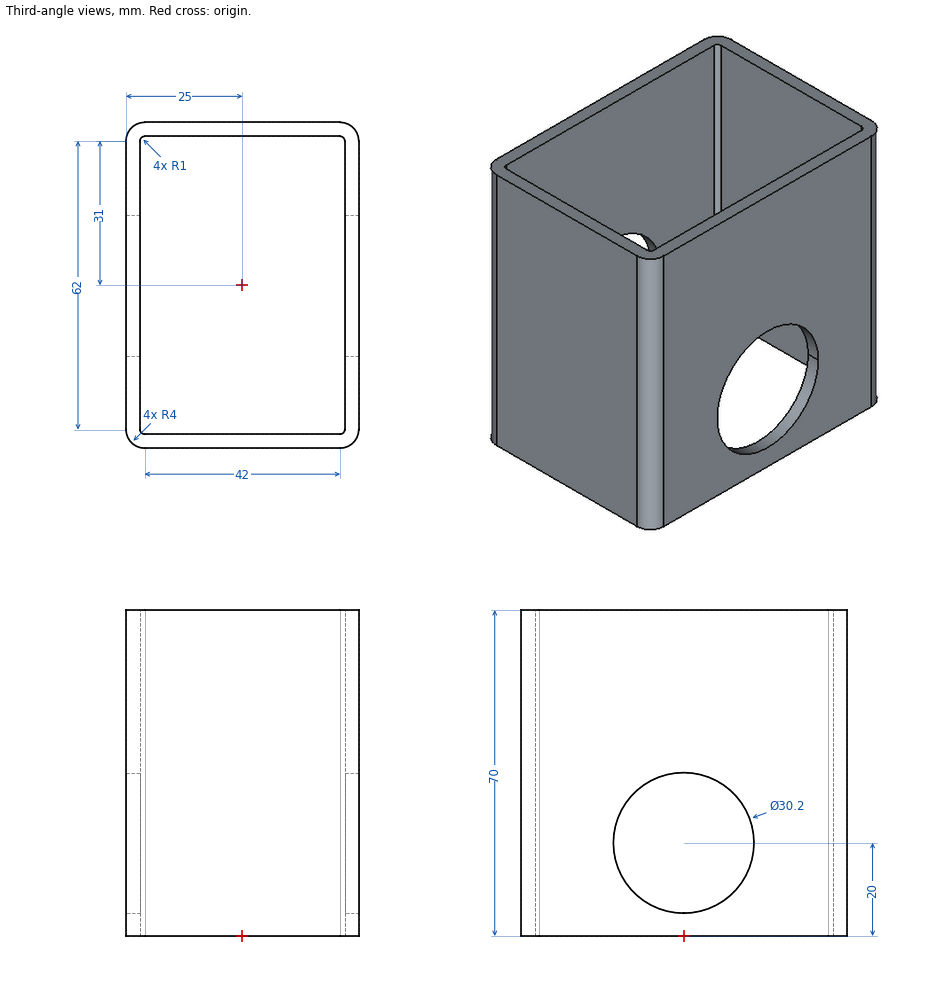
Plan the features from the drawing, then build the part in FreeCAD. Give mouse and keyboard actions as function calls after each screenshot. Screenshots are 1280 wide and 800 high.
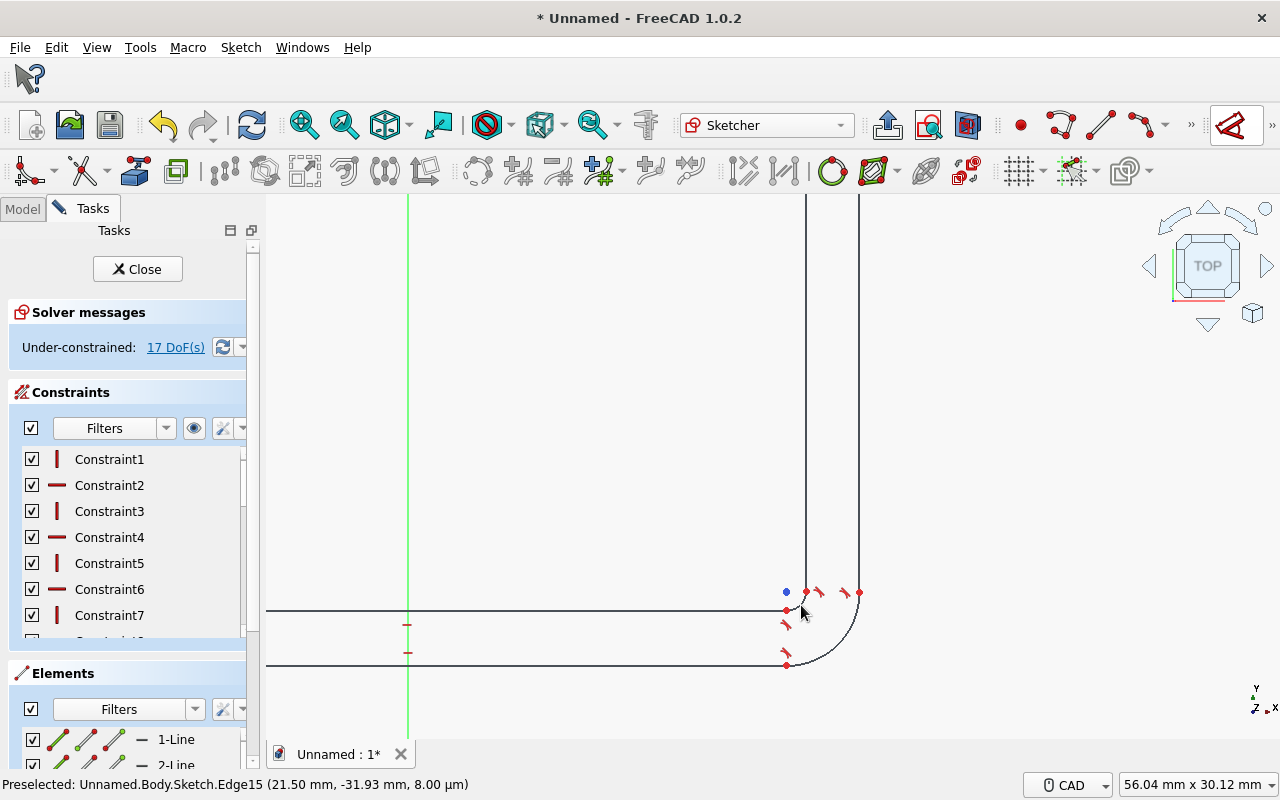
click(559, 611)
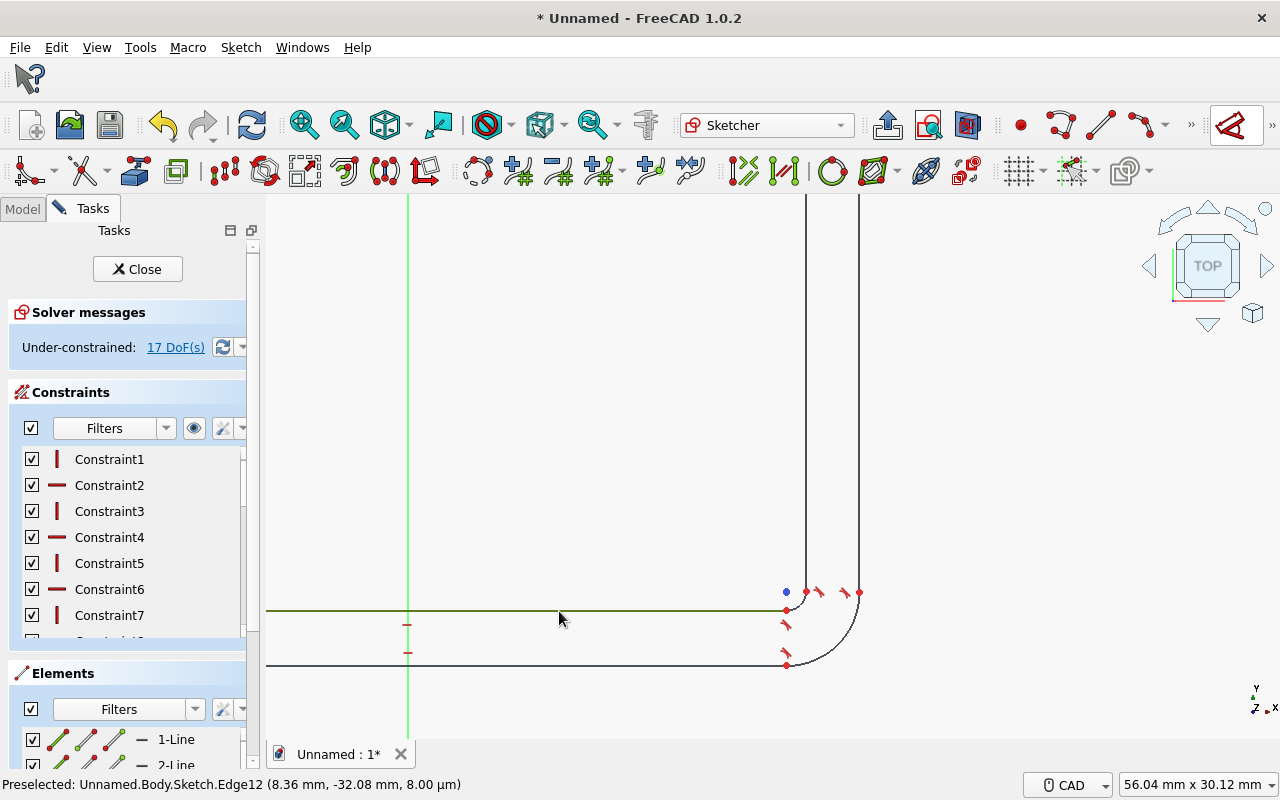
scroll(802, 609, down, 7)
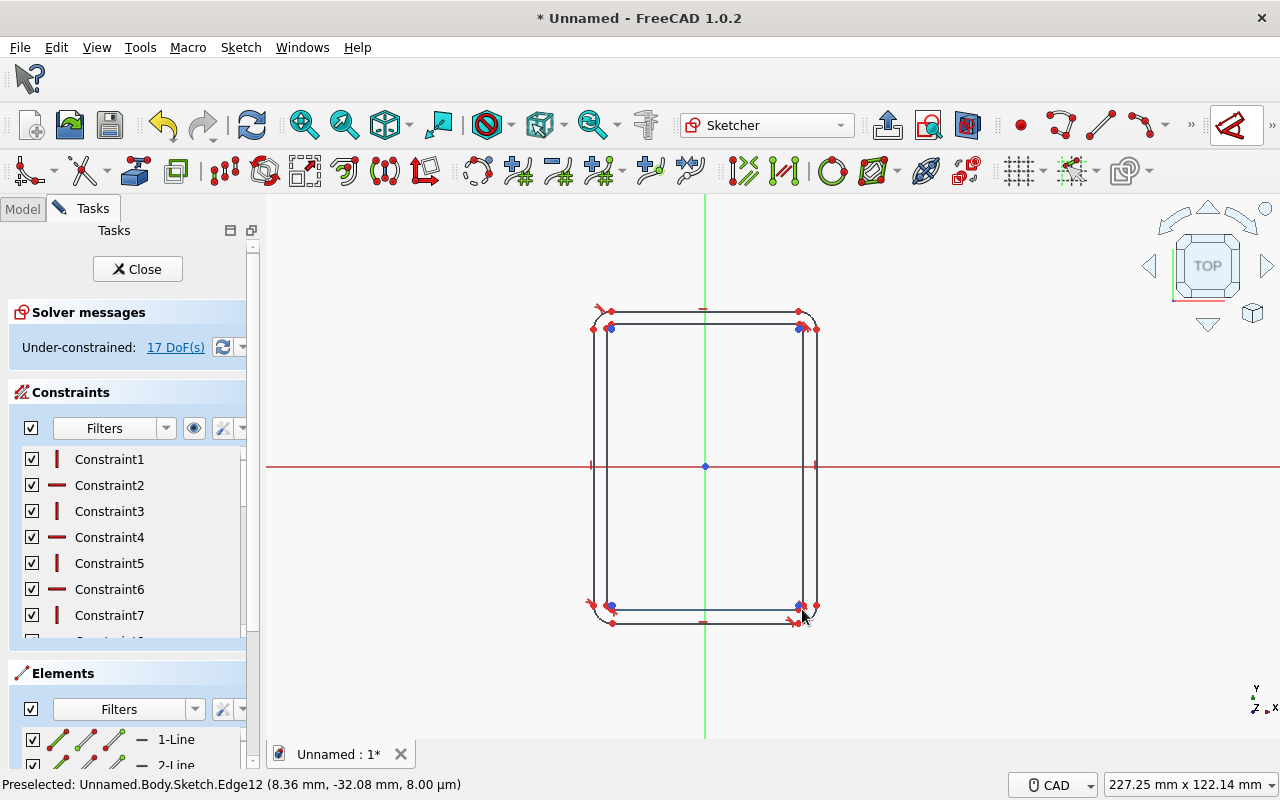
scroll(607, 607, up, 10)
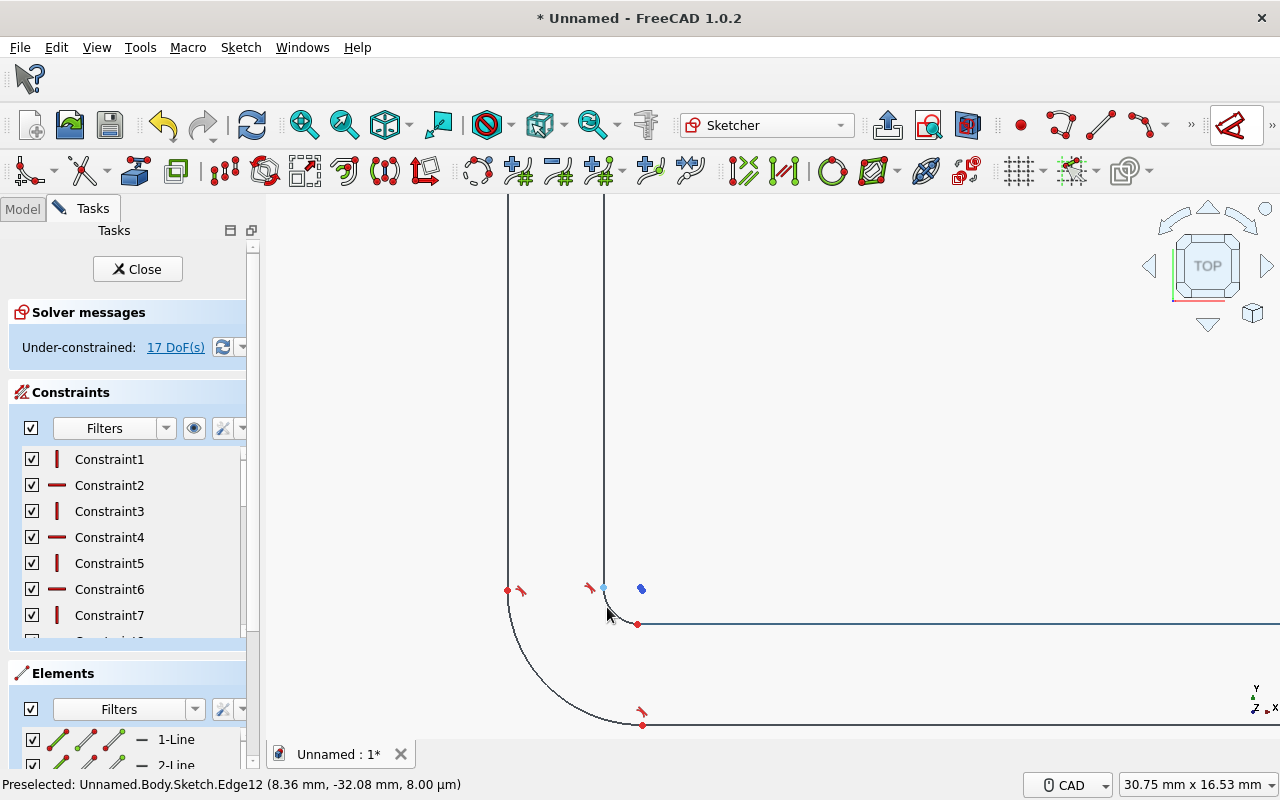
click(607, 603)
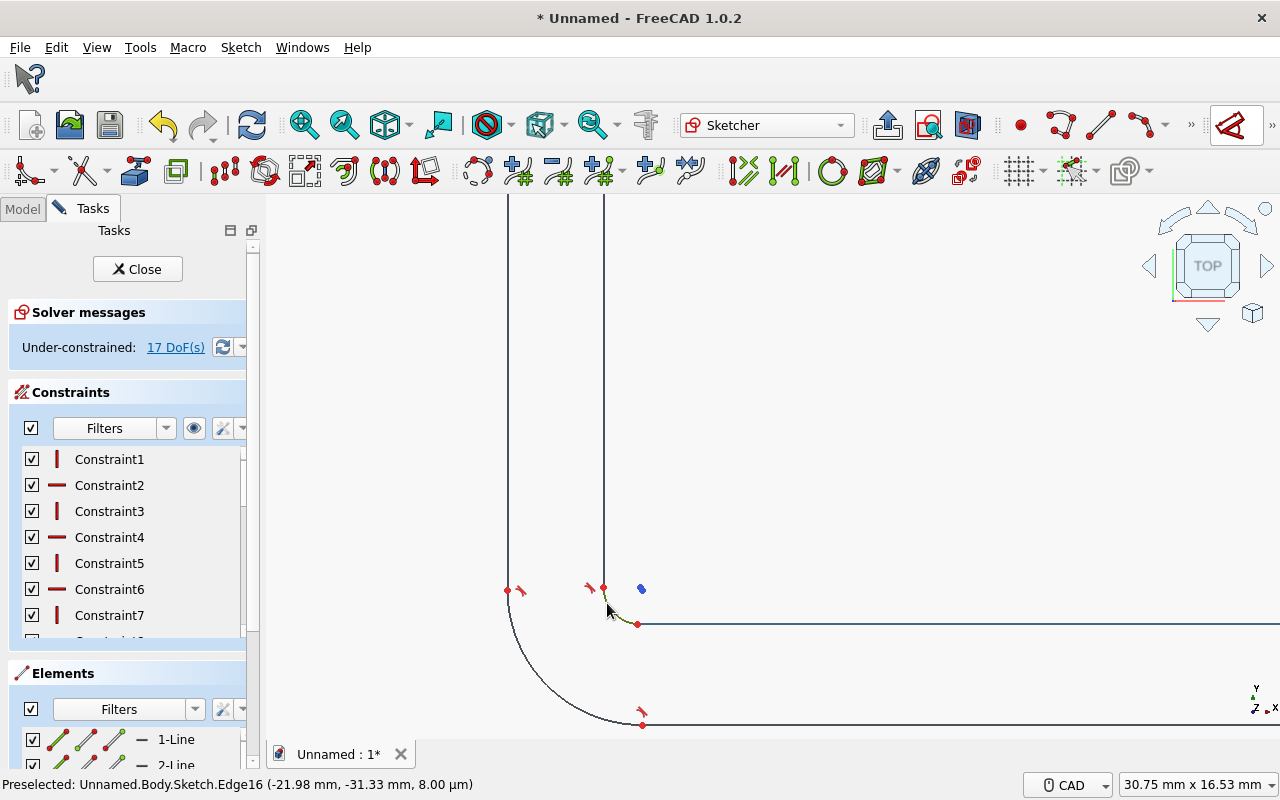
key(t)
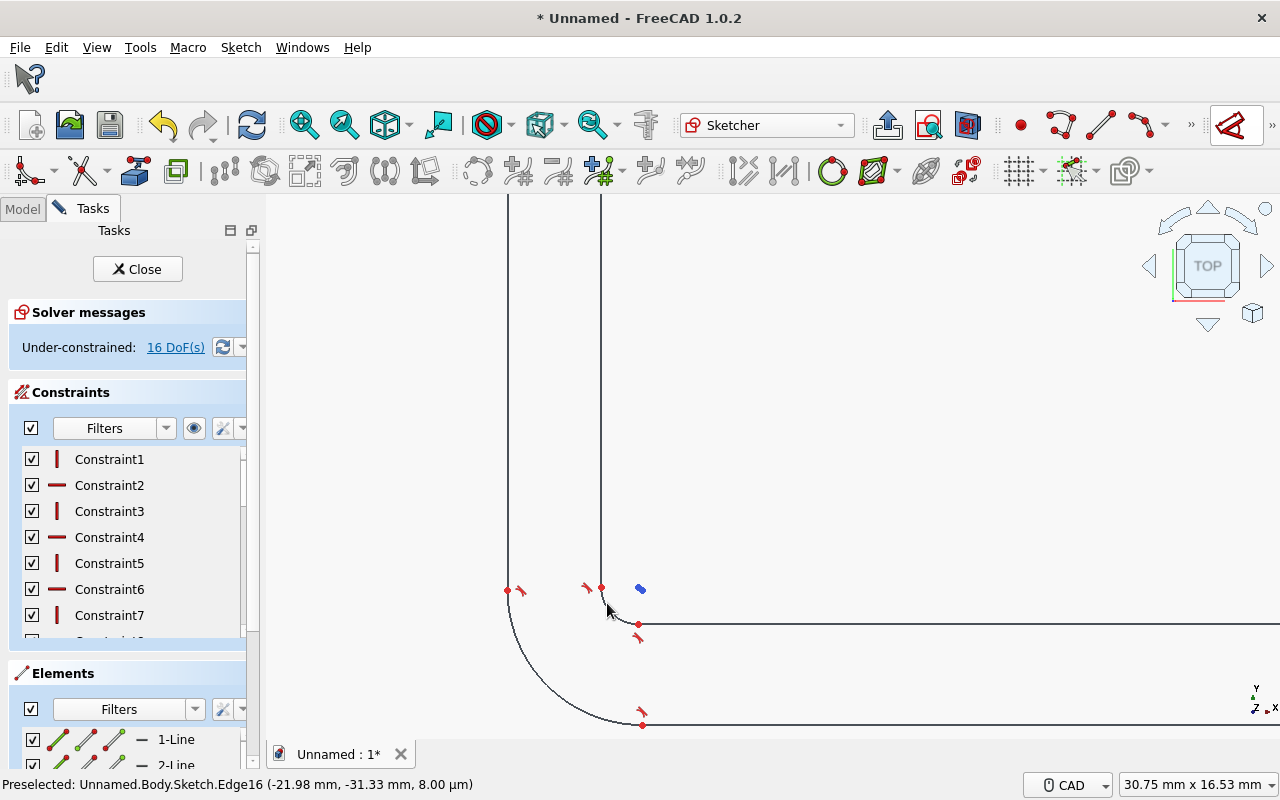
scroll(607, 607, down, 10)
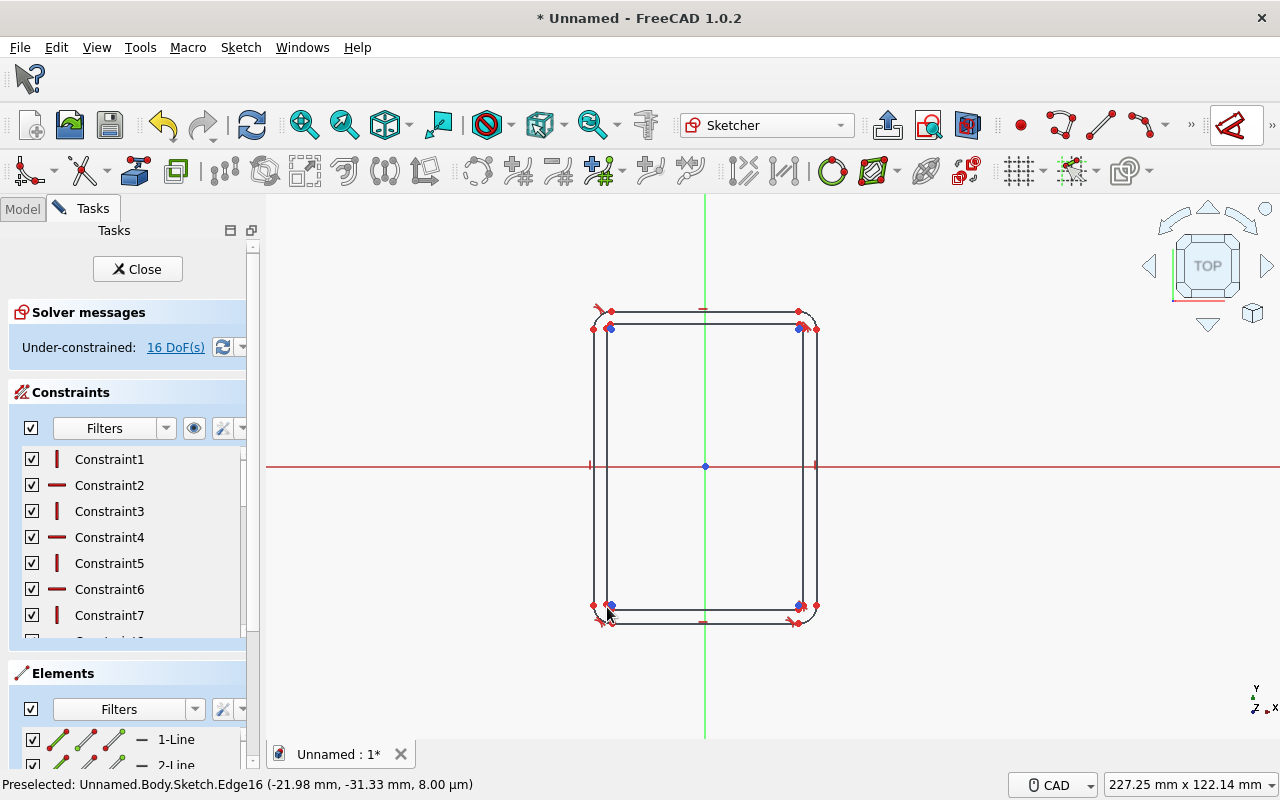
scroll(604, 314, up, 3)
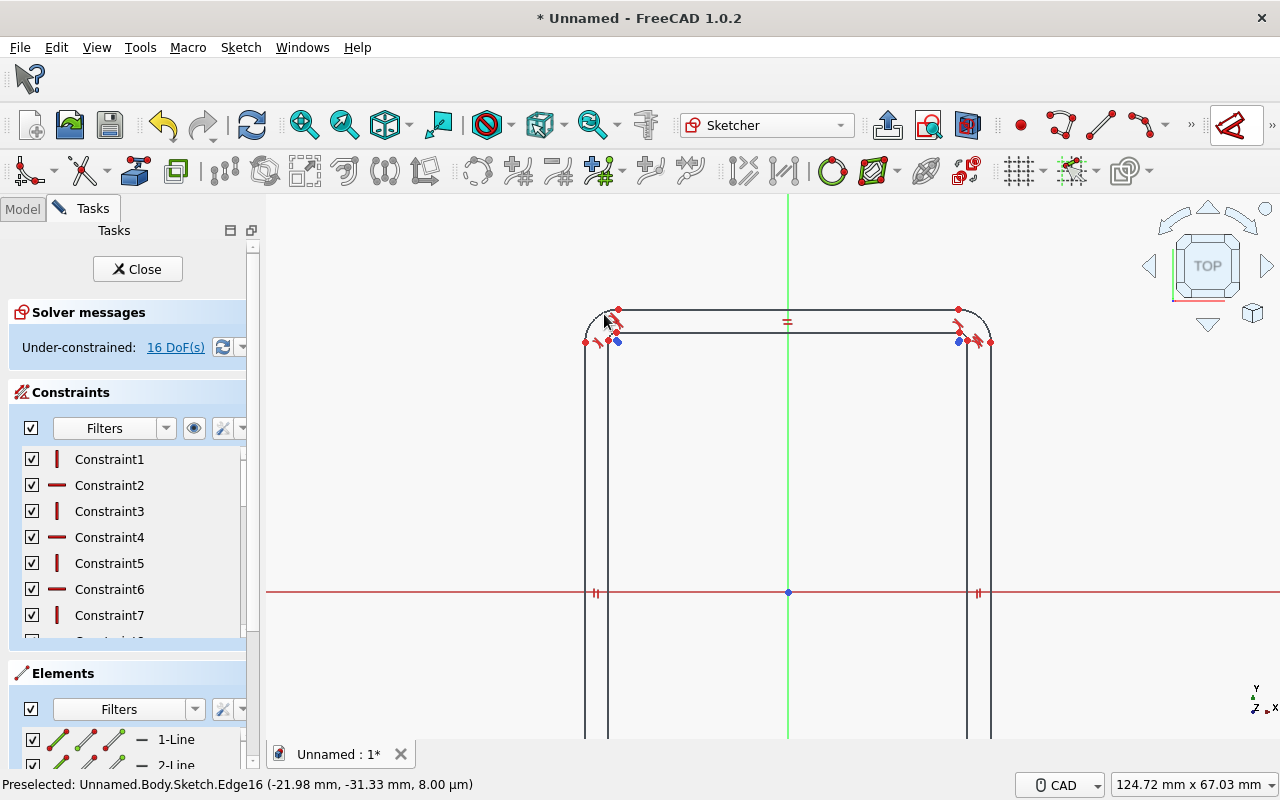
click(603, 313)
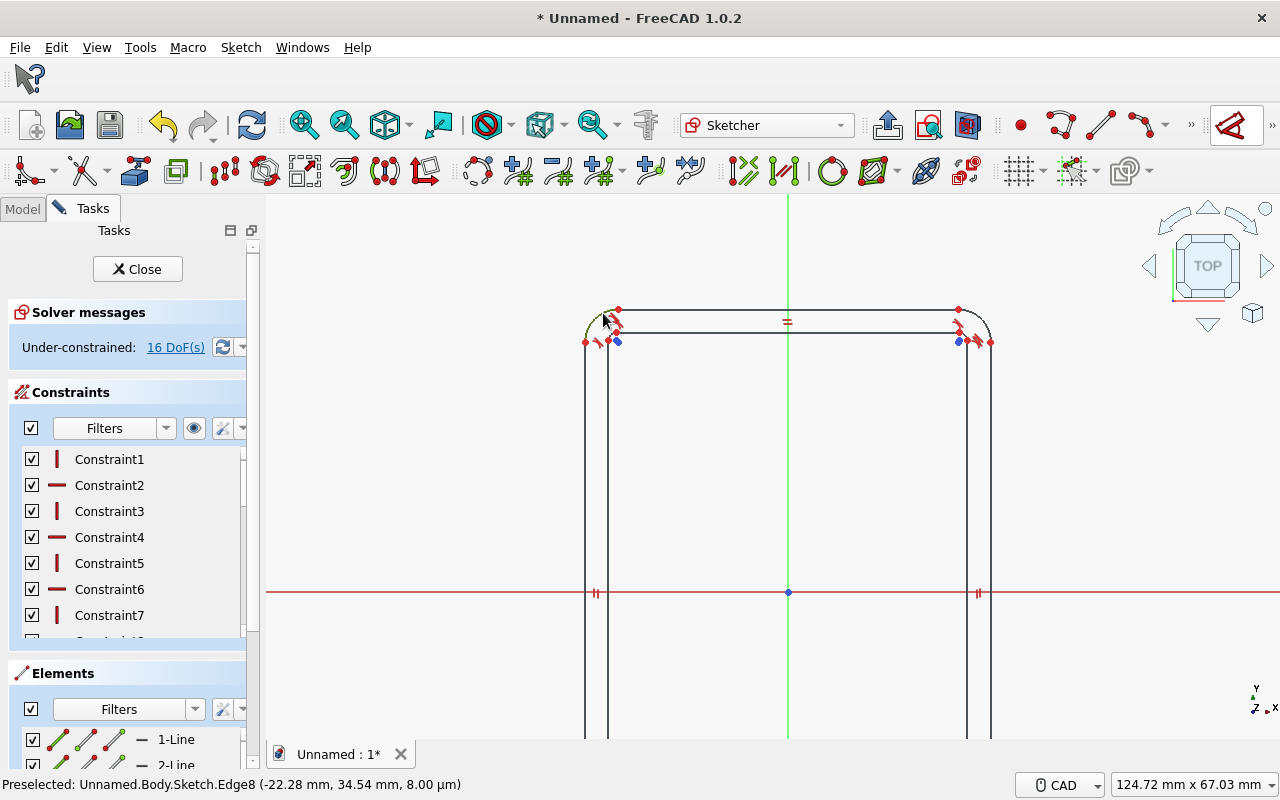
scroll(611, 335, up, 5)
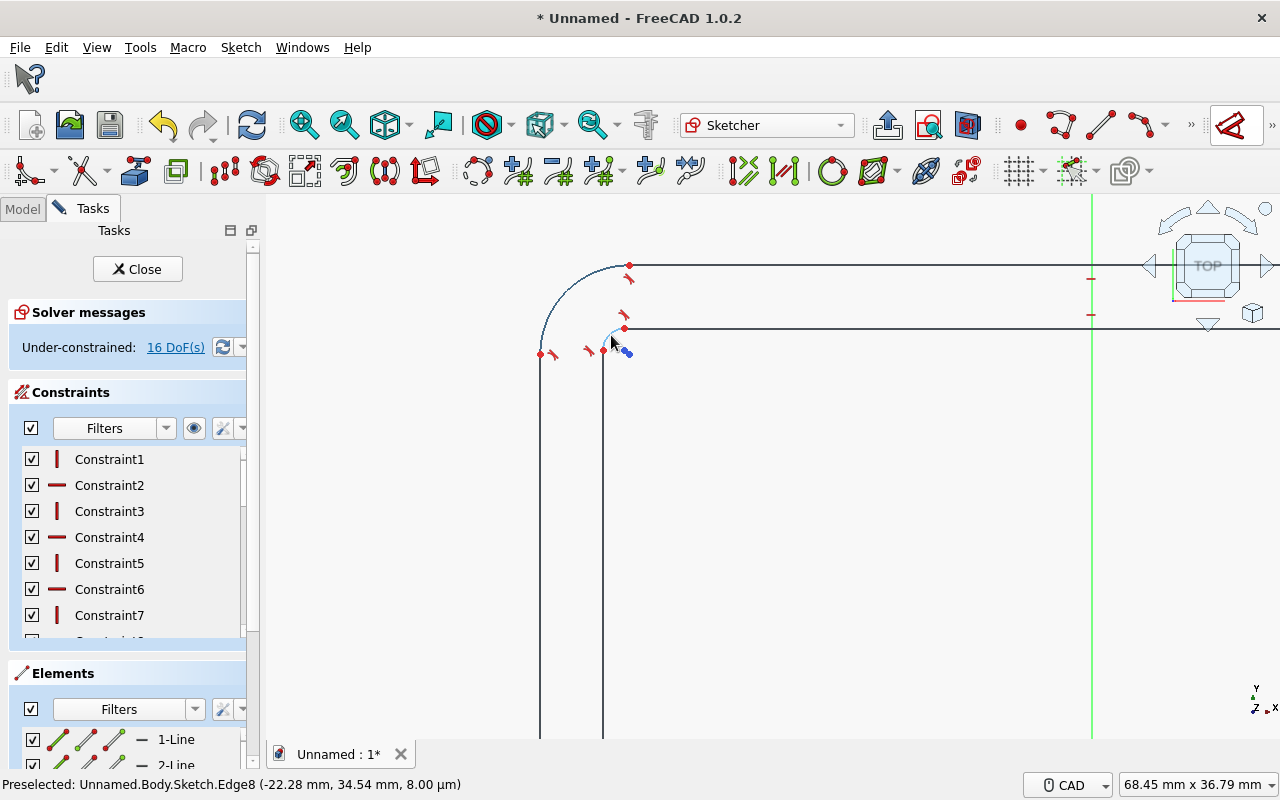
click(609, 335)